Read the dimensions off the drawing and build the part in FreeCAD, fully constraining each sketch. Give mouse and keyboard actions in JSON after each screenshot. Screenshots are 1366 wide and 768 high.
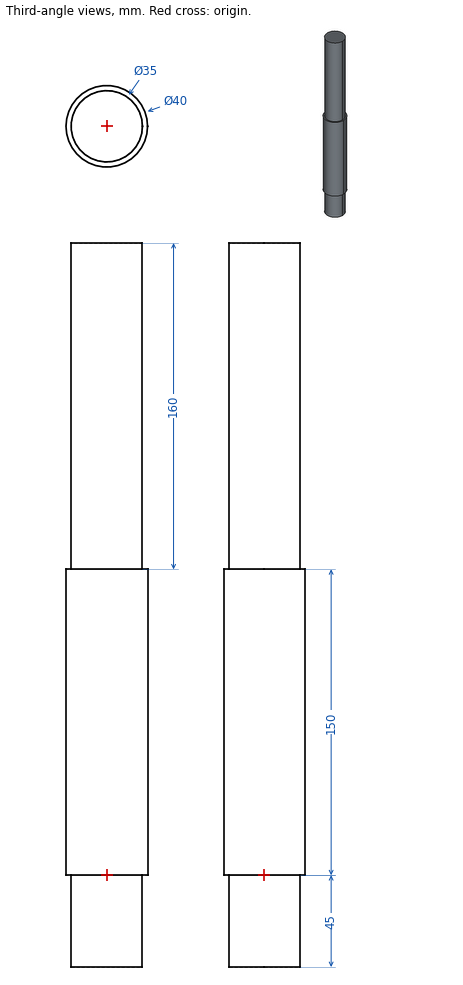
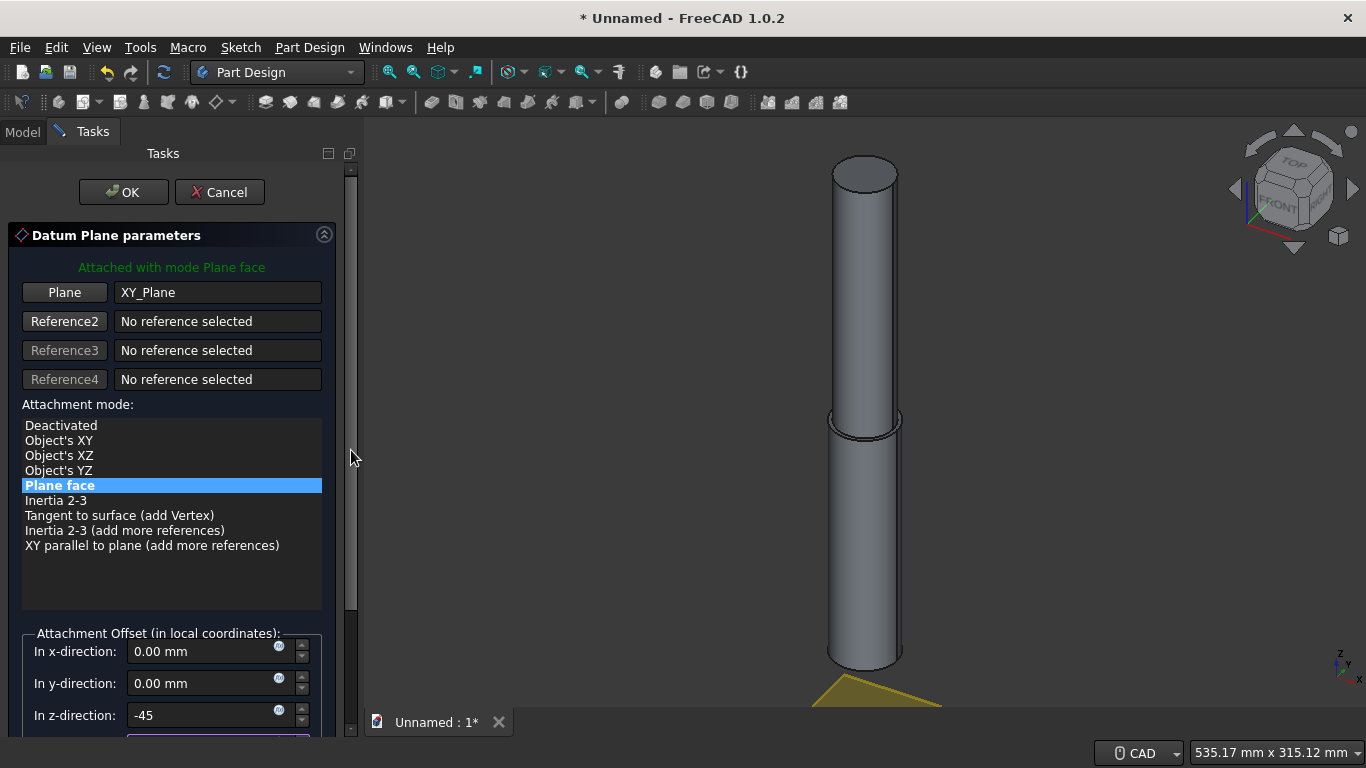
{"action": "left_click", "coordinate": [124, 192]}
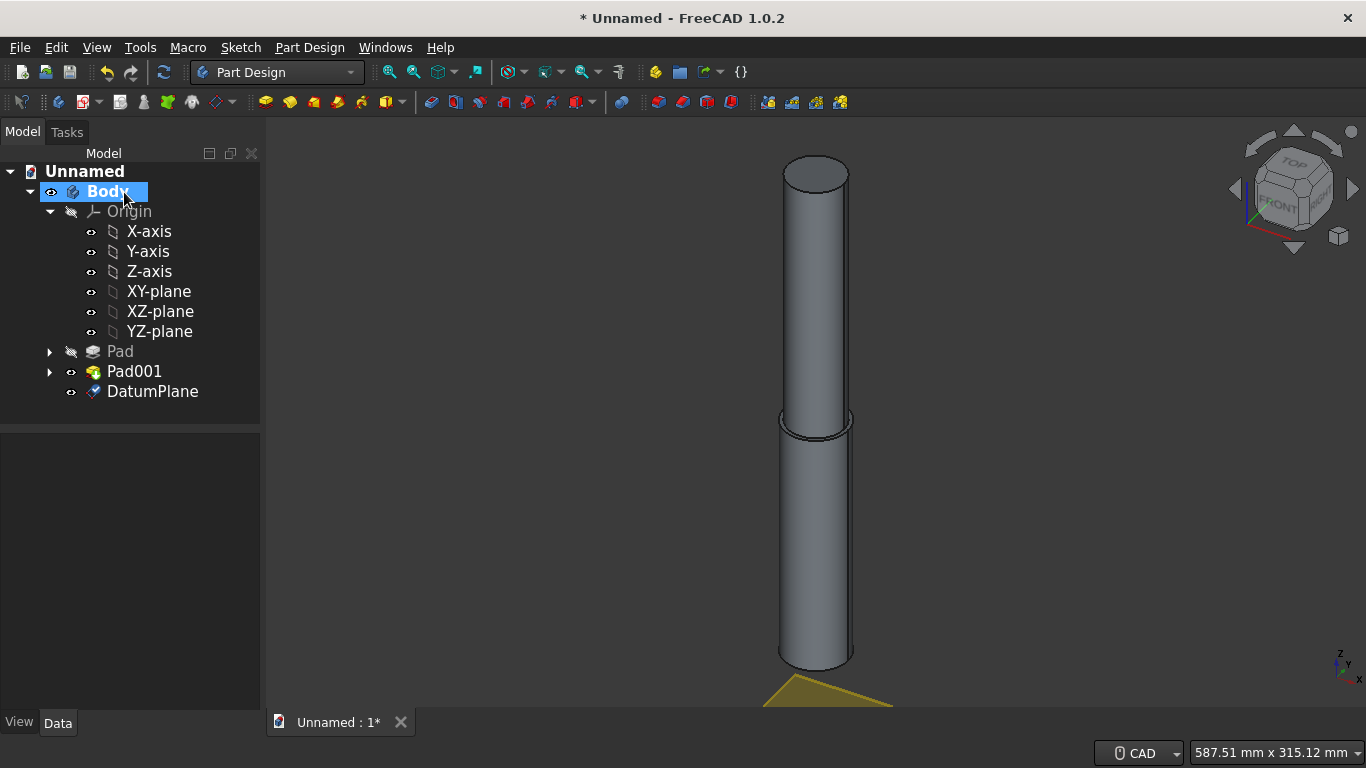
{"action": "left_click", "coordinate": [116, 392]}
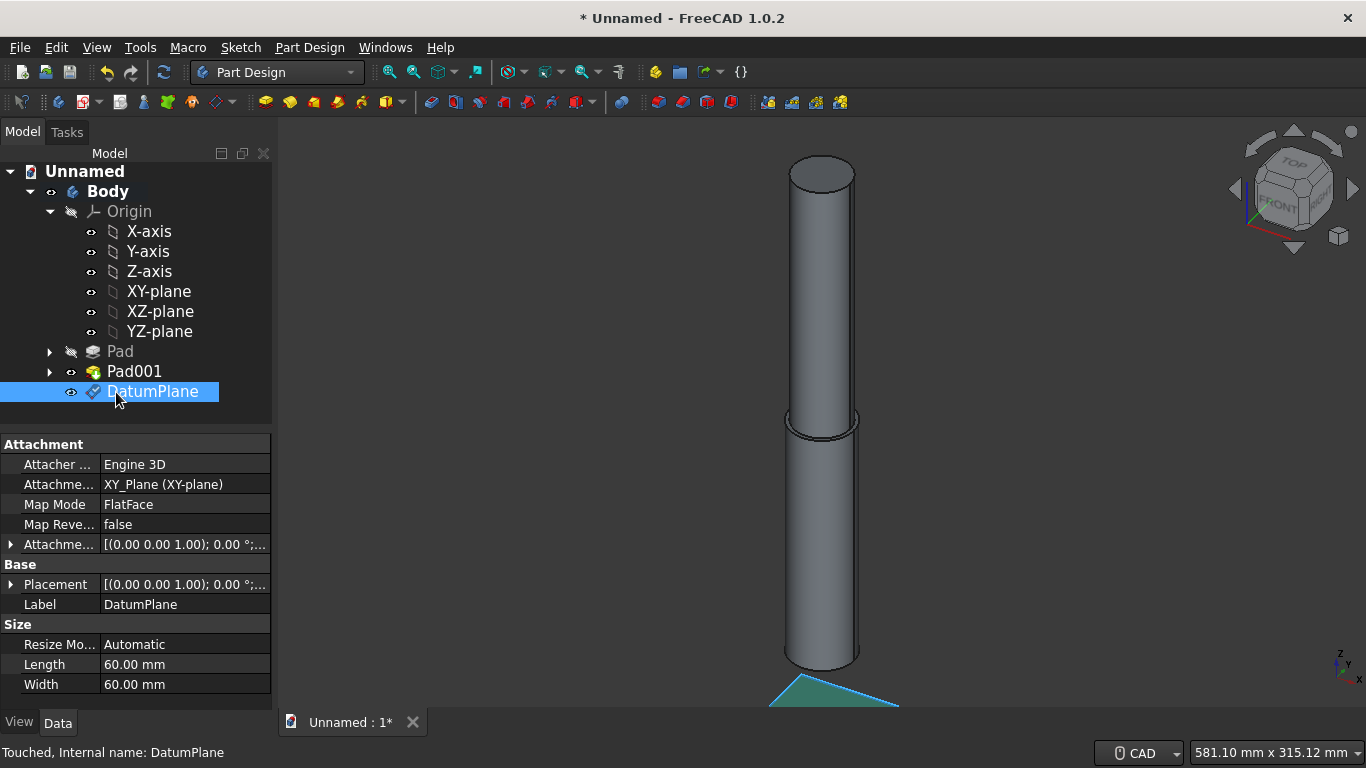
{"action": "left_click", "coordinate": [84, 102]}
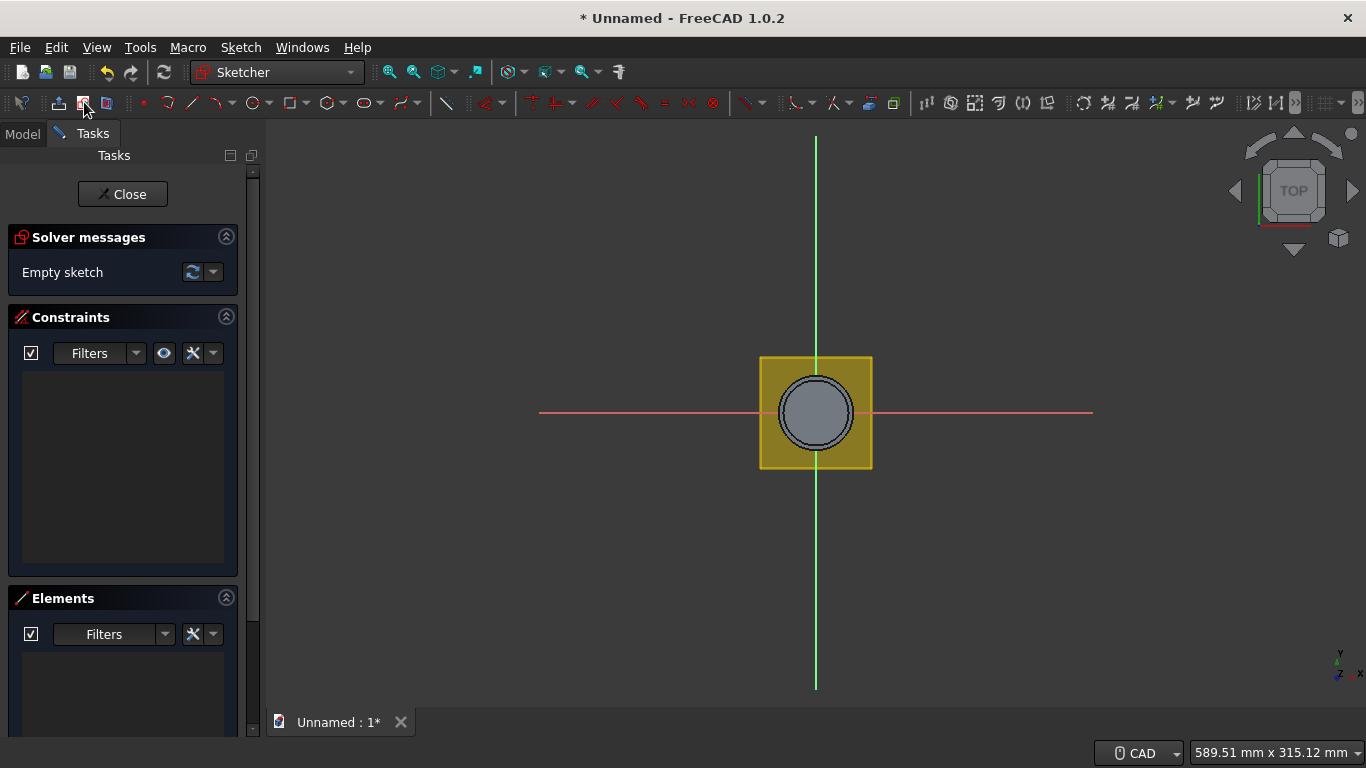
{"action": "key", "text": "q s"}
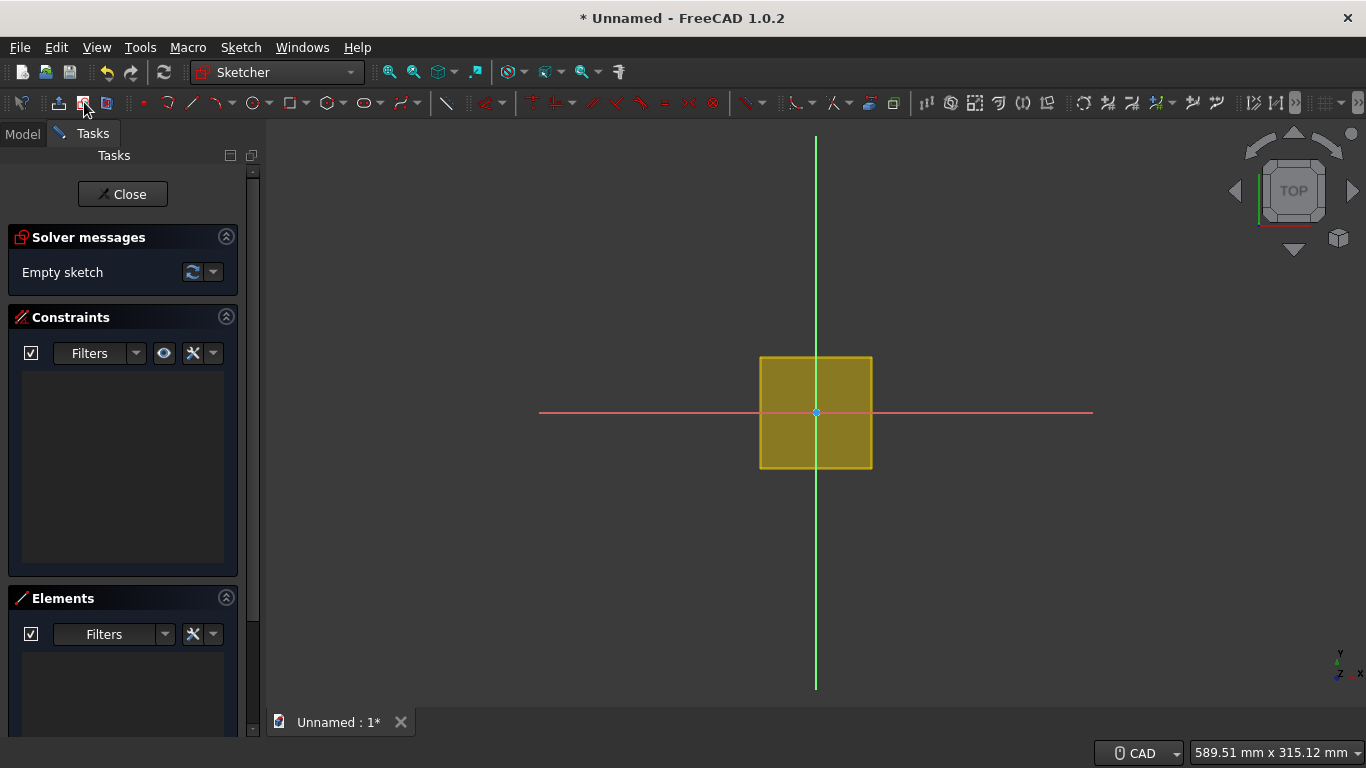
{"action": "scroll", "coordinate": [830, 413], "scroll_direction": "up", "scroll_amount": 9}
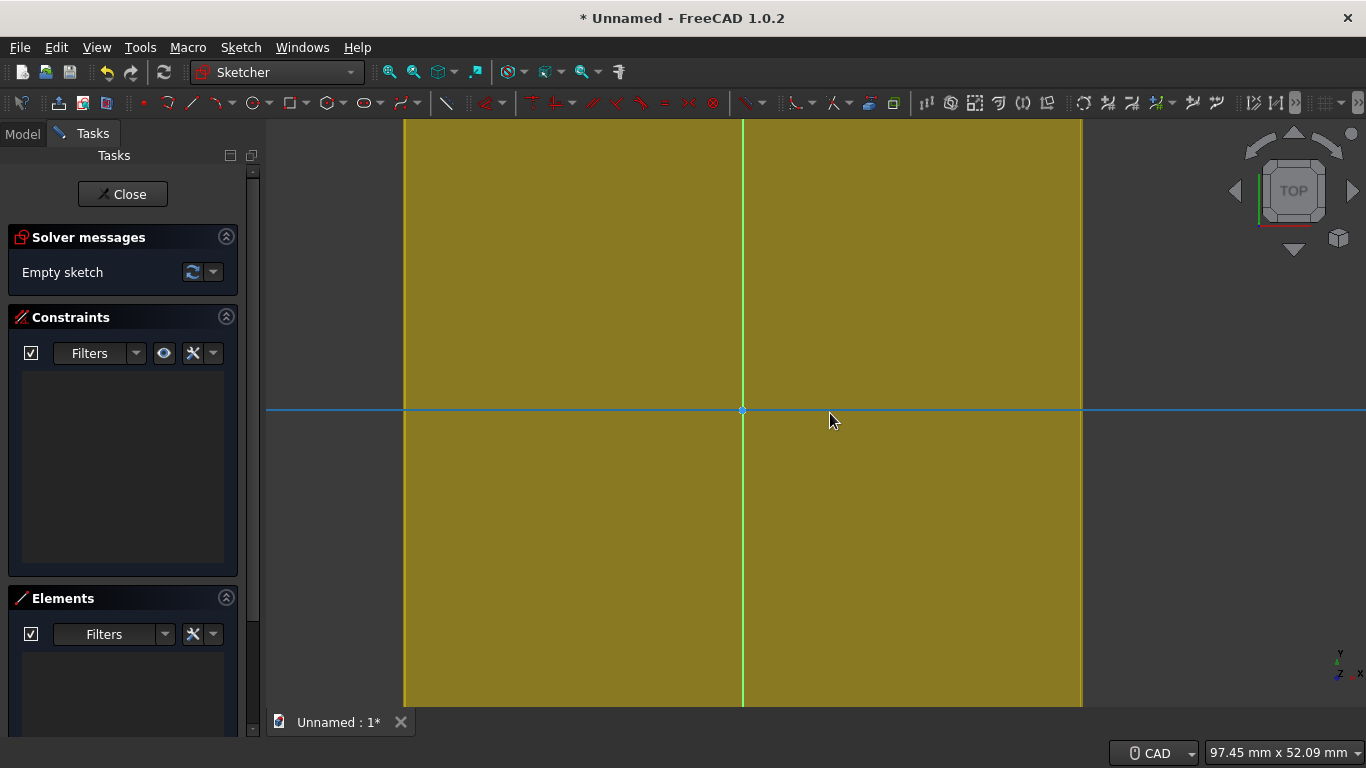
{"action": "key", "text": "g c"}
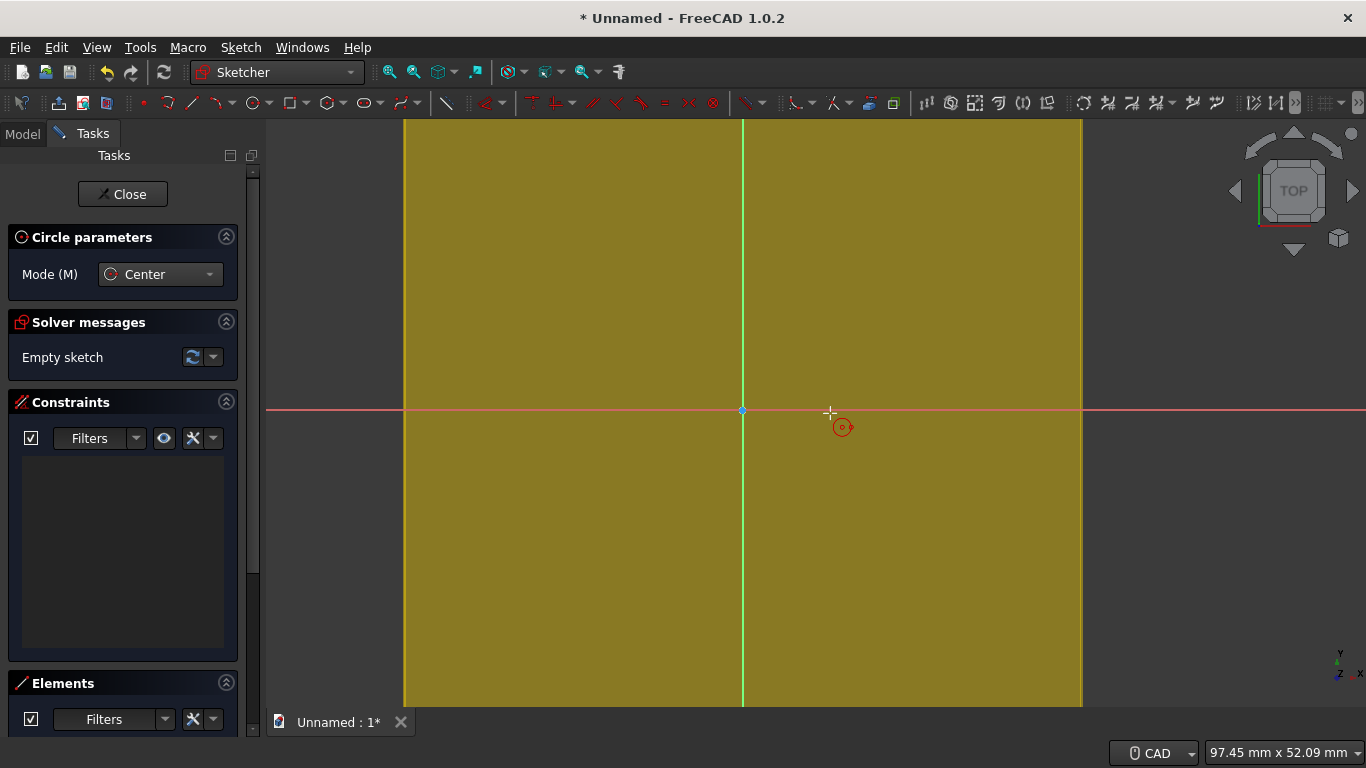
{"action": "left_click", "coordinate": [743, 410]}
{"action": "mouse_move", "coordinate": [882, 271]}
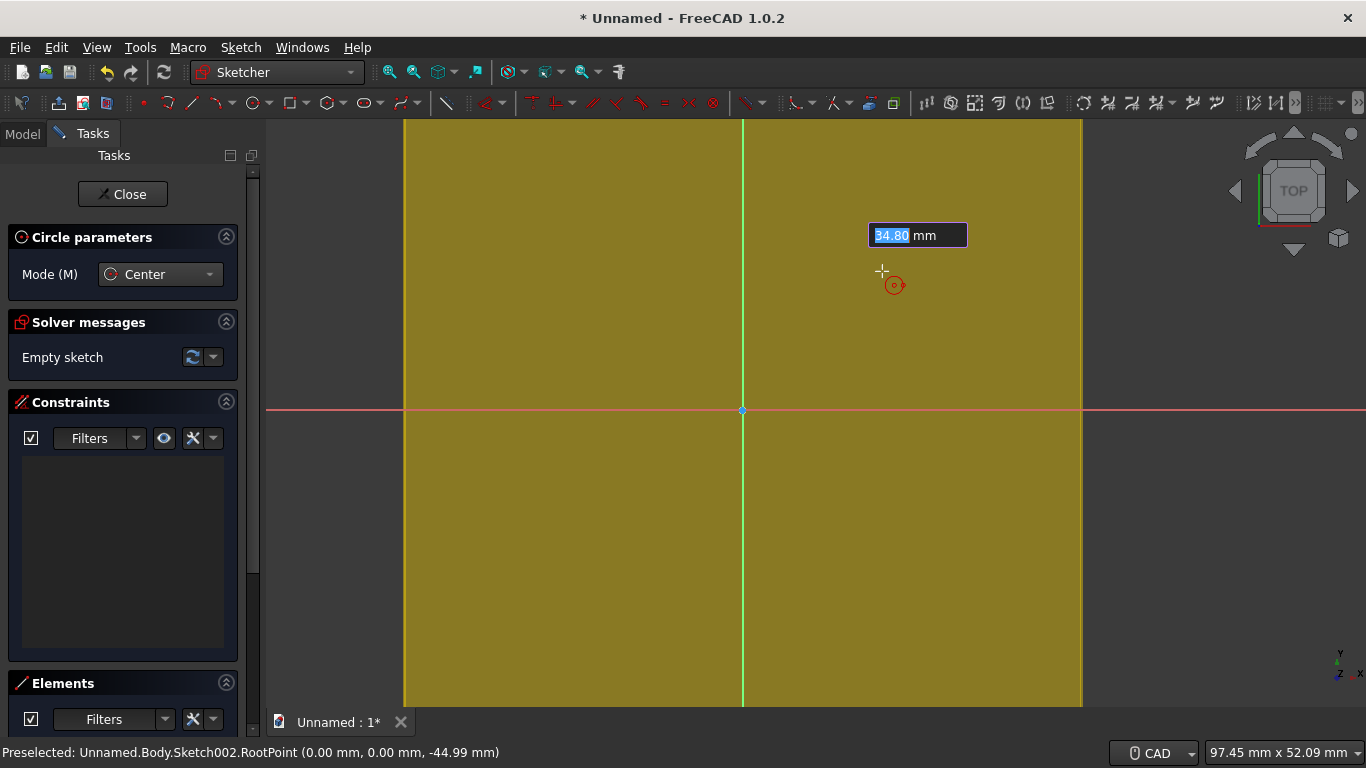
{"action": "type", "text": "35"}
{"action": "key", "text": "Return"}
{"action": "key", "text": "Escape"}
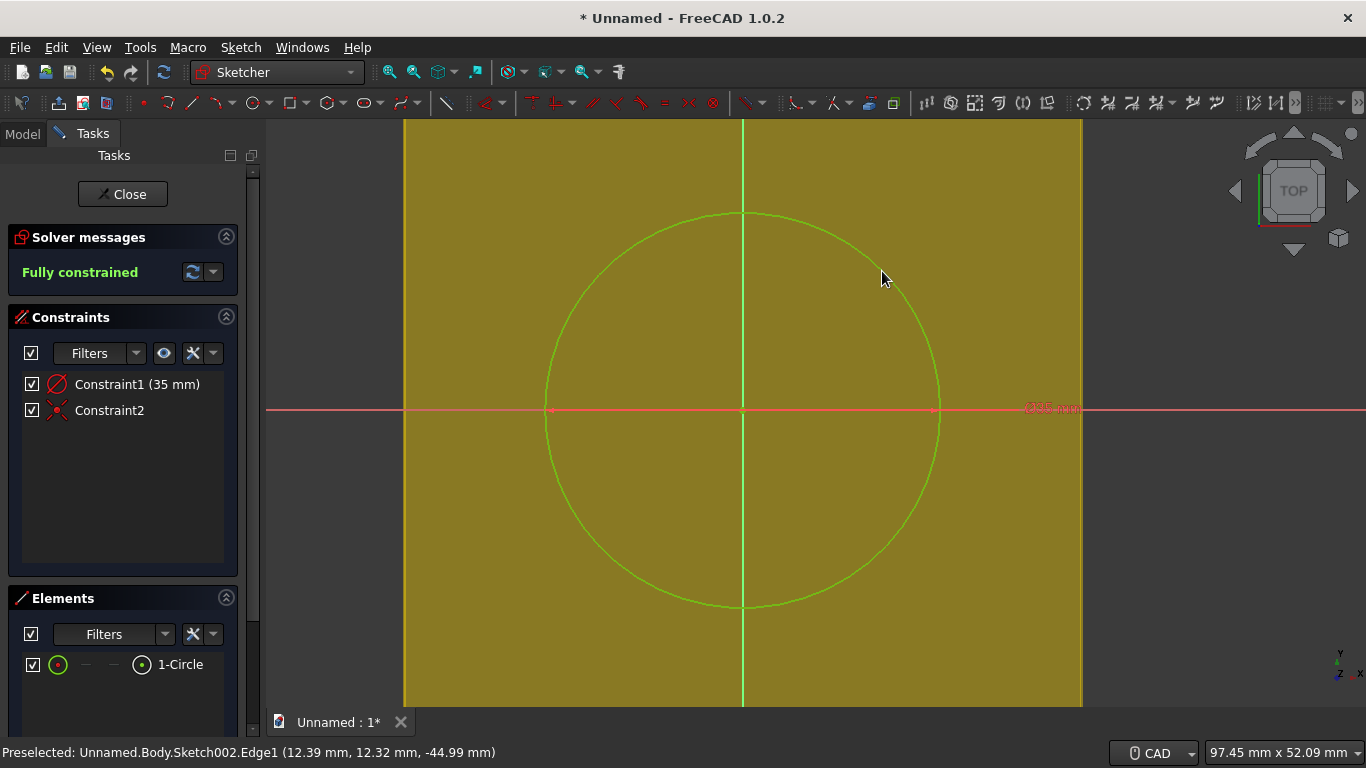
{"action": "left_click", "coordinate": [123, 194]}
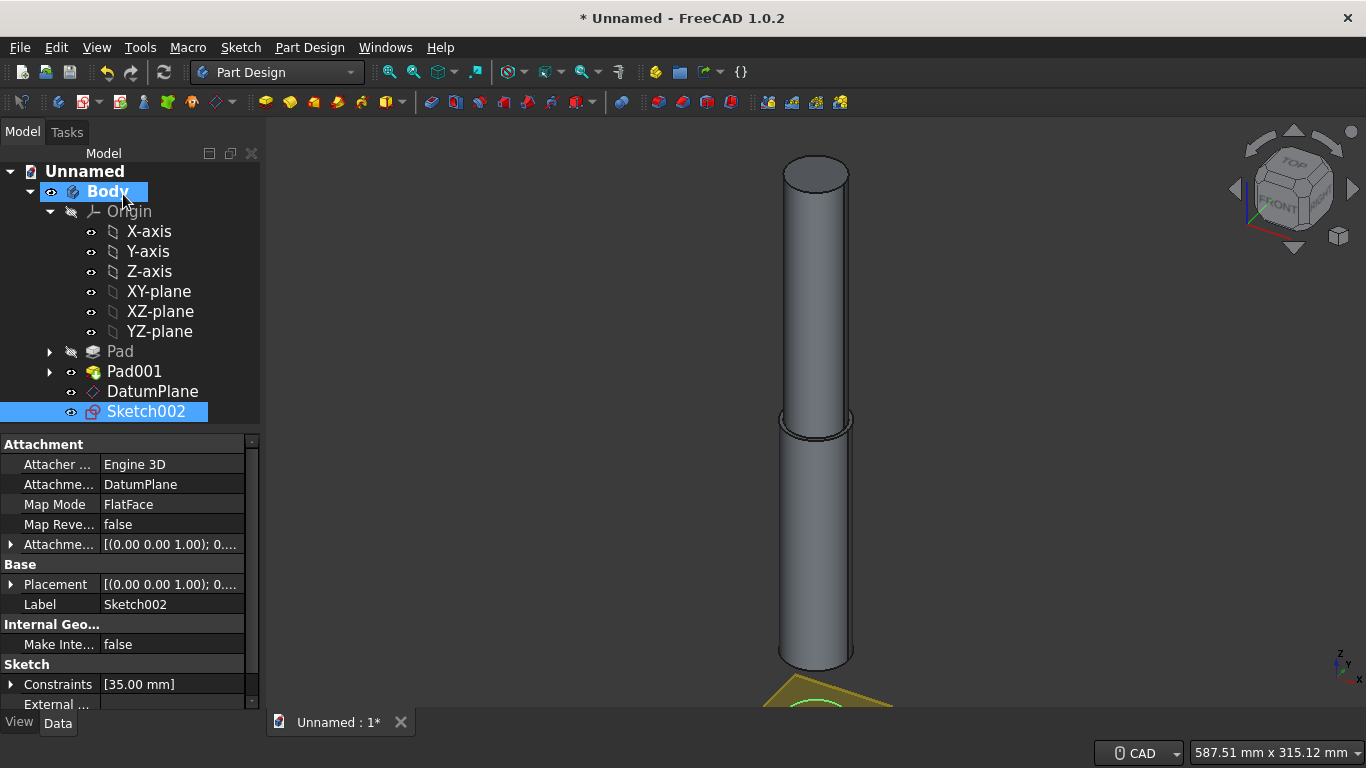
{"action": "left_click", "coordinate": [266, 102]}